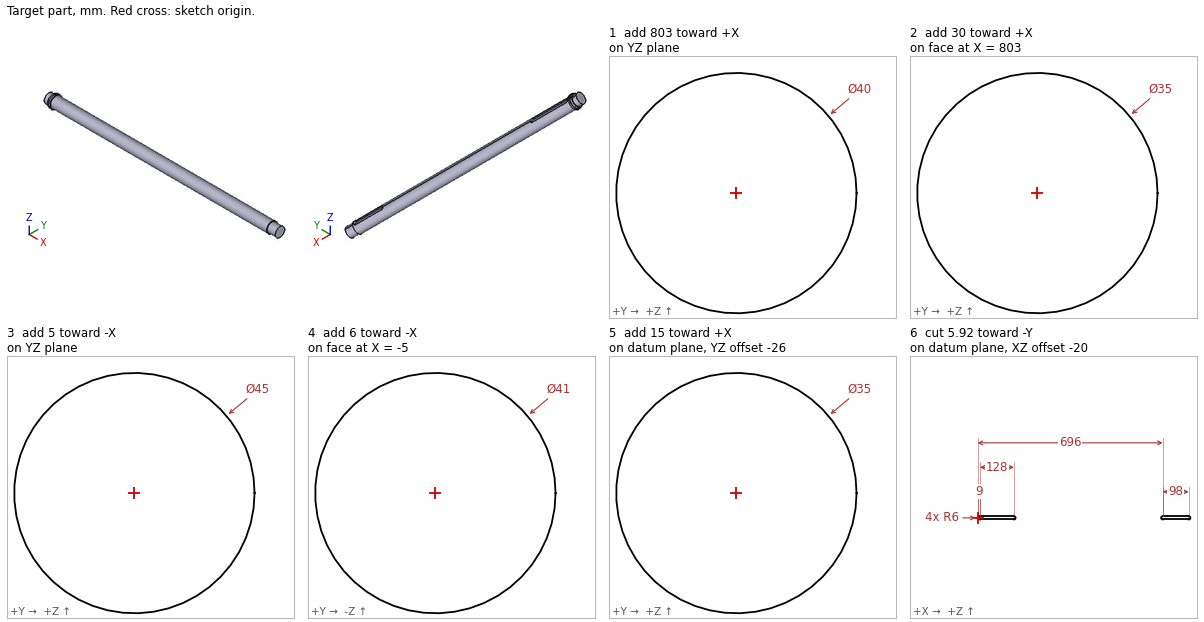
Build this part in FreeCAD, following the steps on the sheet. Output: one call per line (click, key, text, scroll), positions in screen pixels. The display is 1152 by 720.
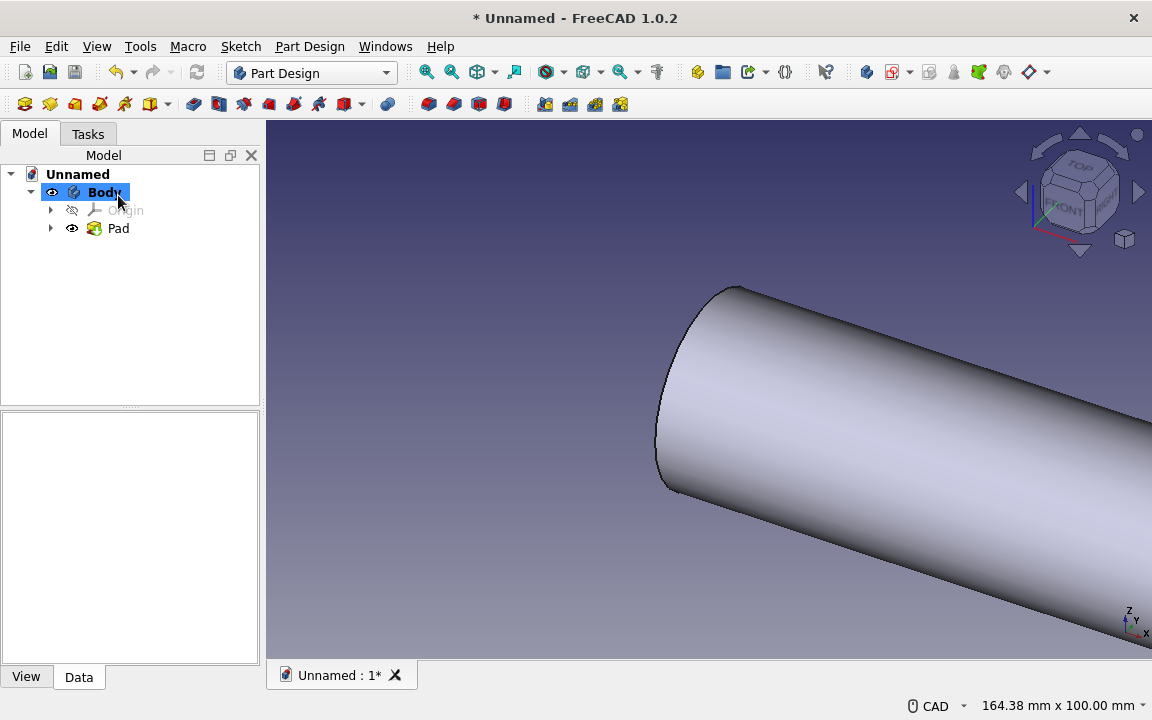
click(427, 72)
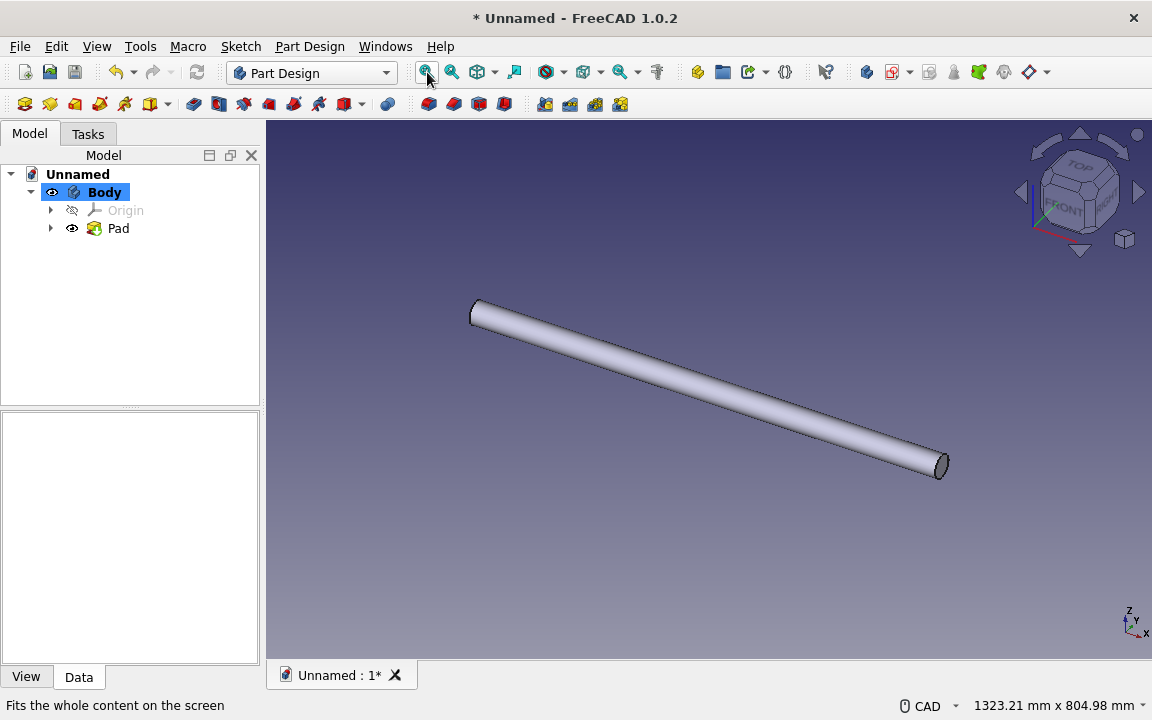
key(0)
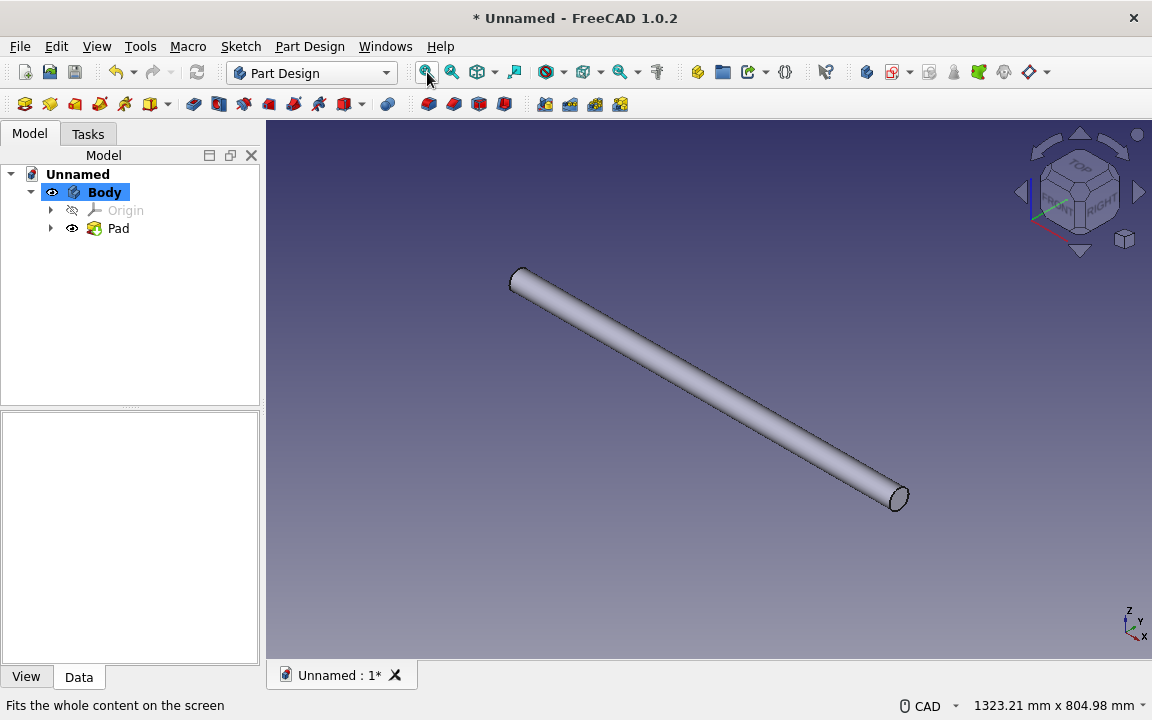
click(902, 497)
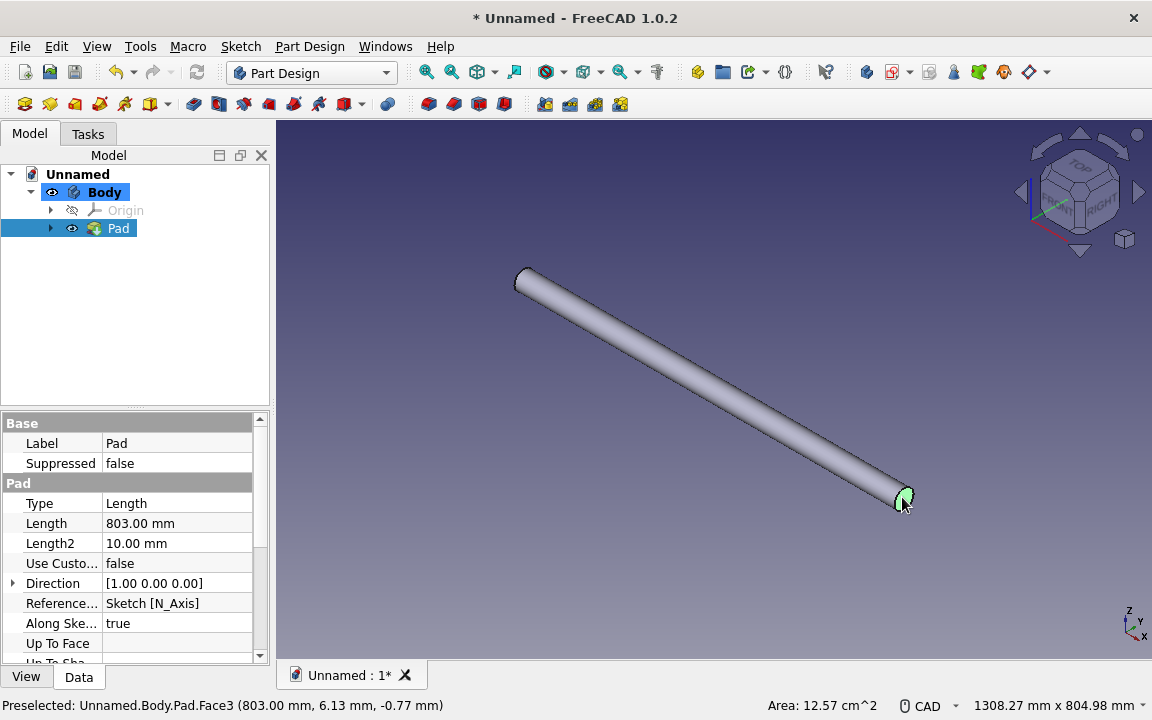
click(892, 72)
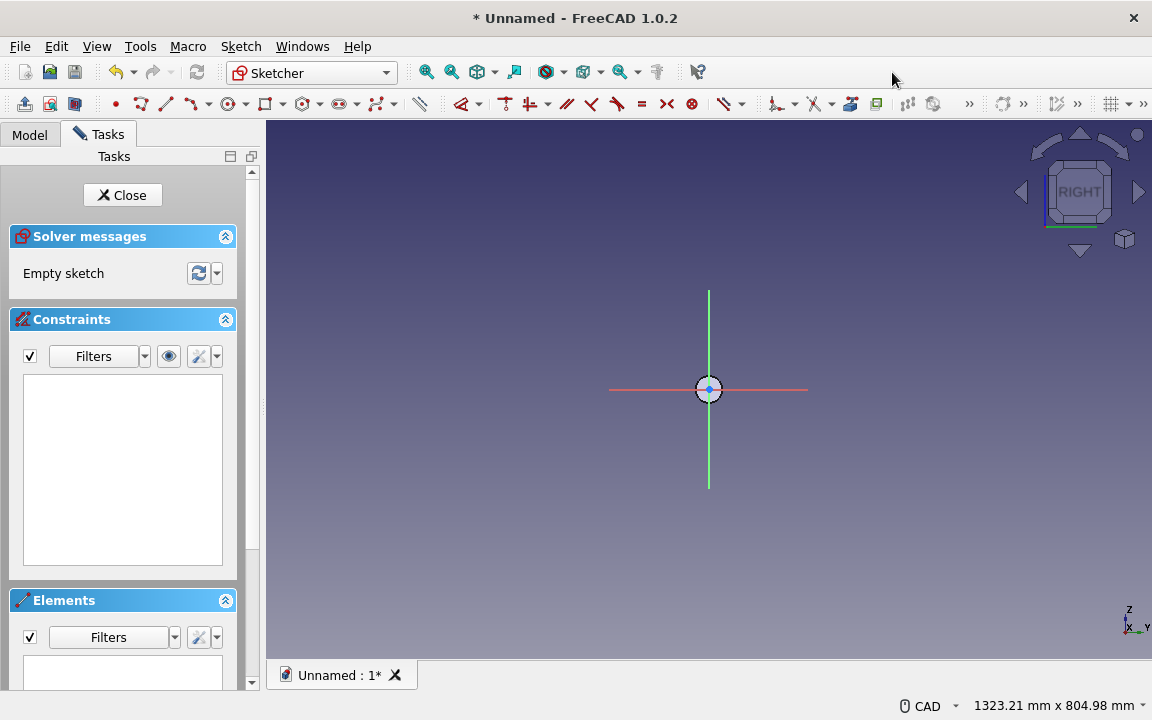
scroll(714, 389, up, 13)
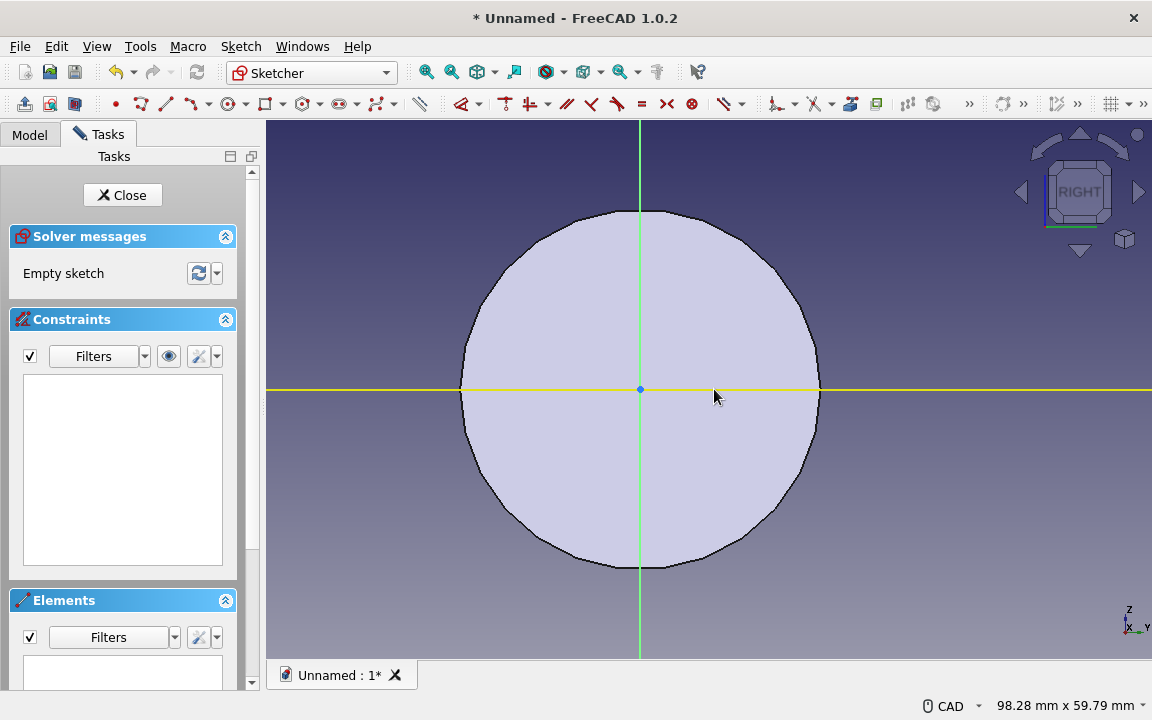
click(228, 104)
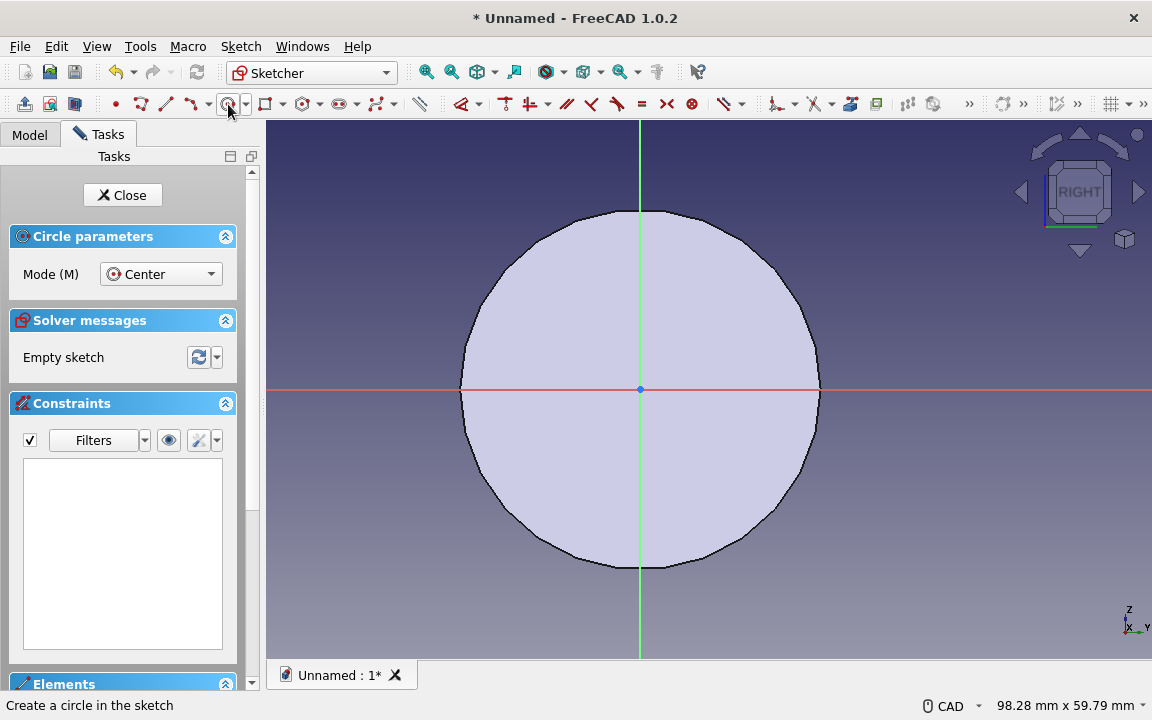
click(640, 389)
move(752, 278)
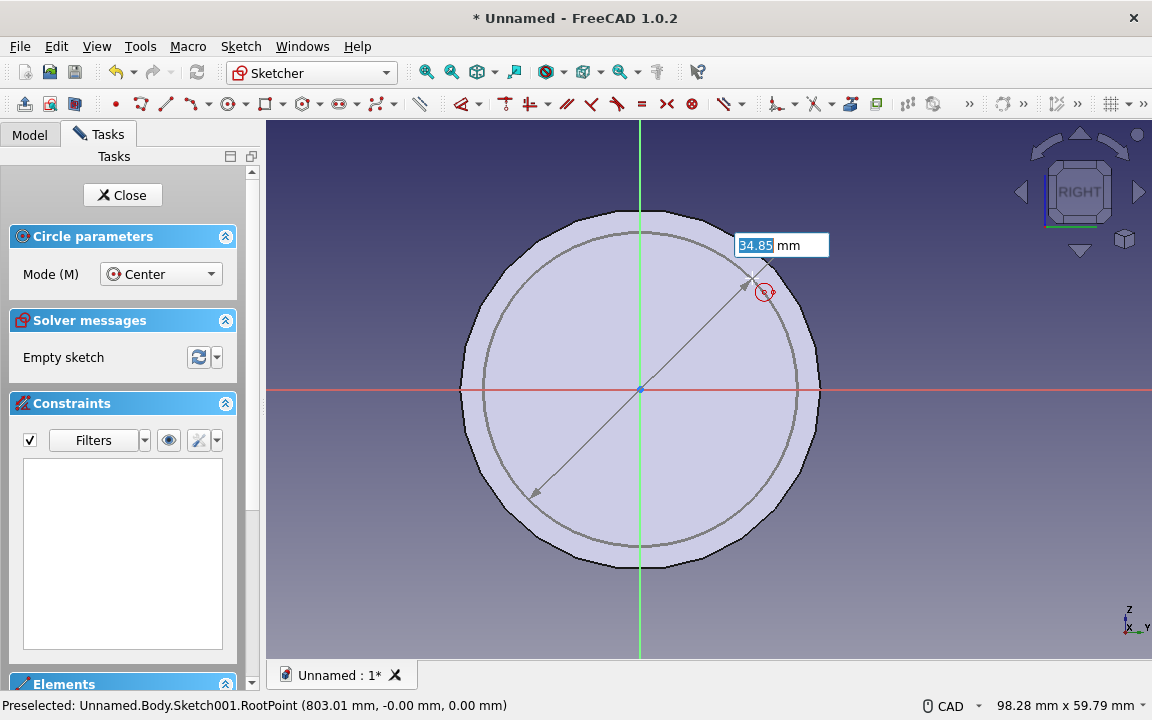
text(35)
key(Return)
key(Escape)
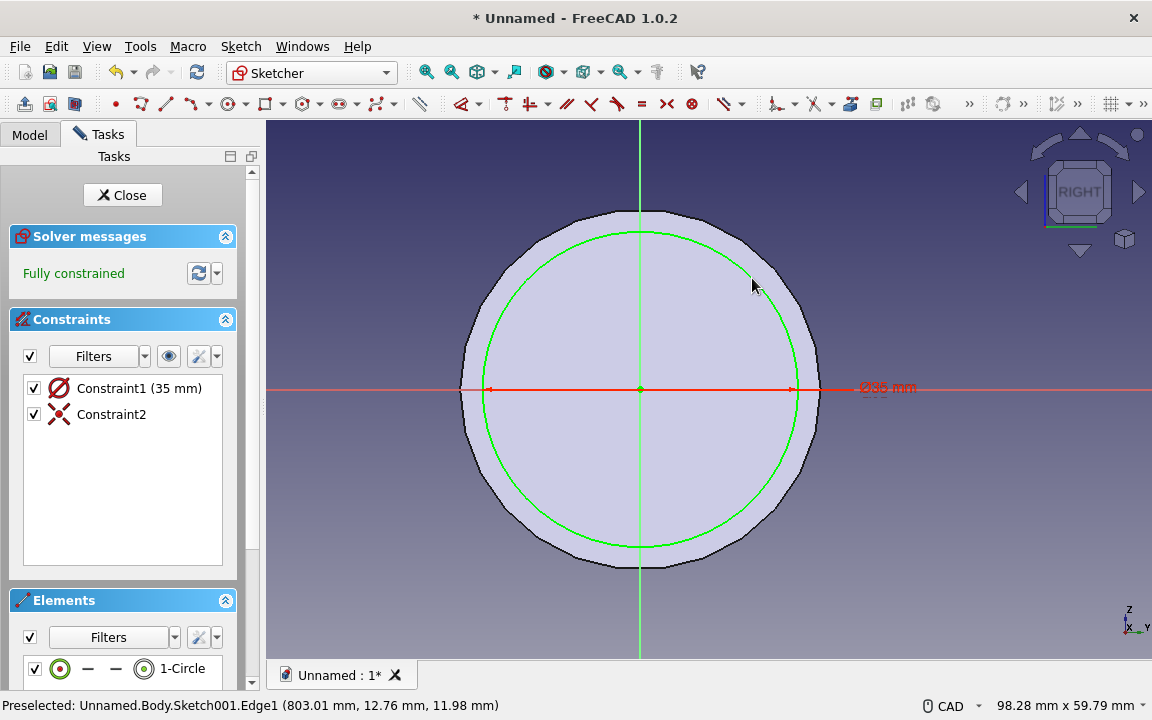
click(123, 195)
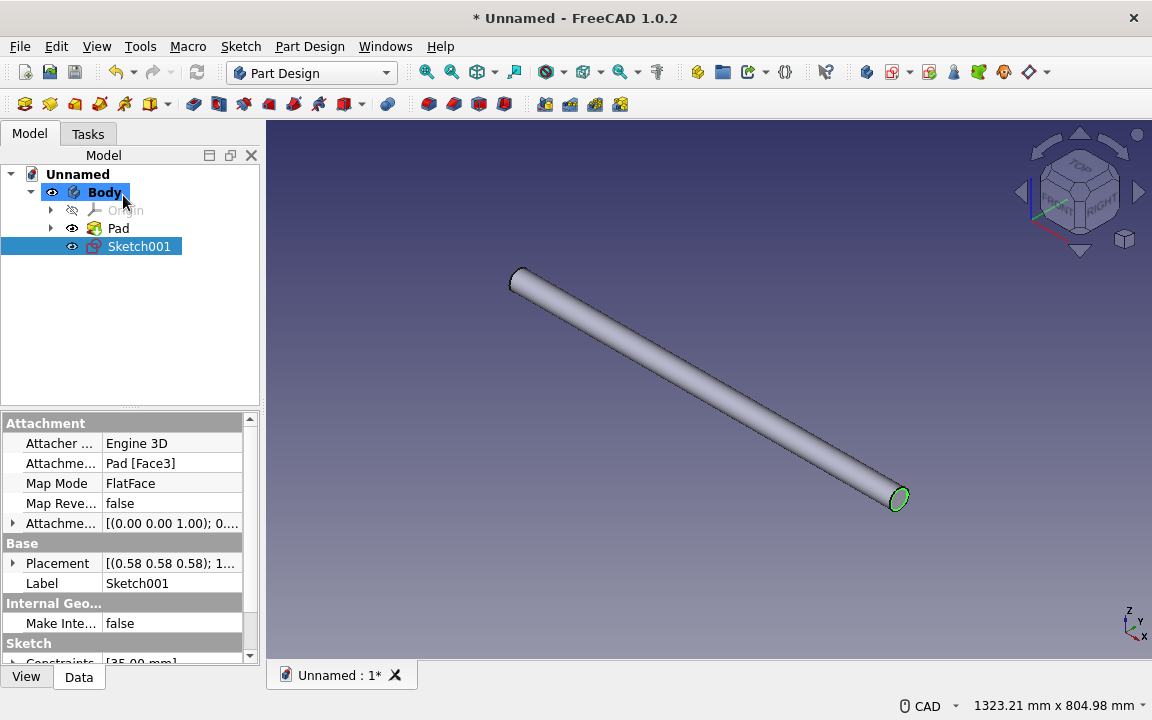
click(25, 104)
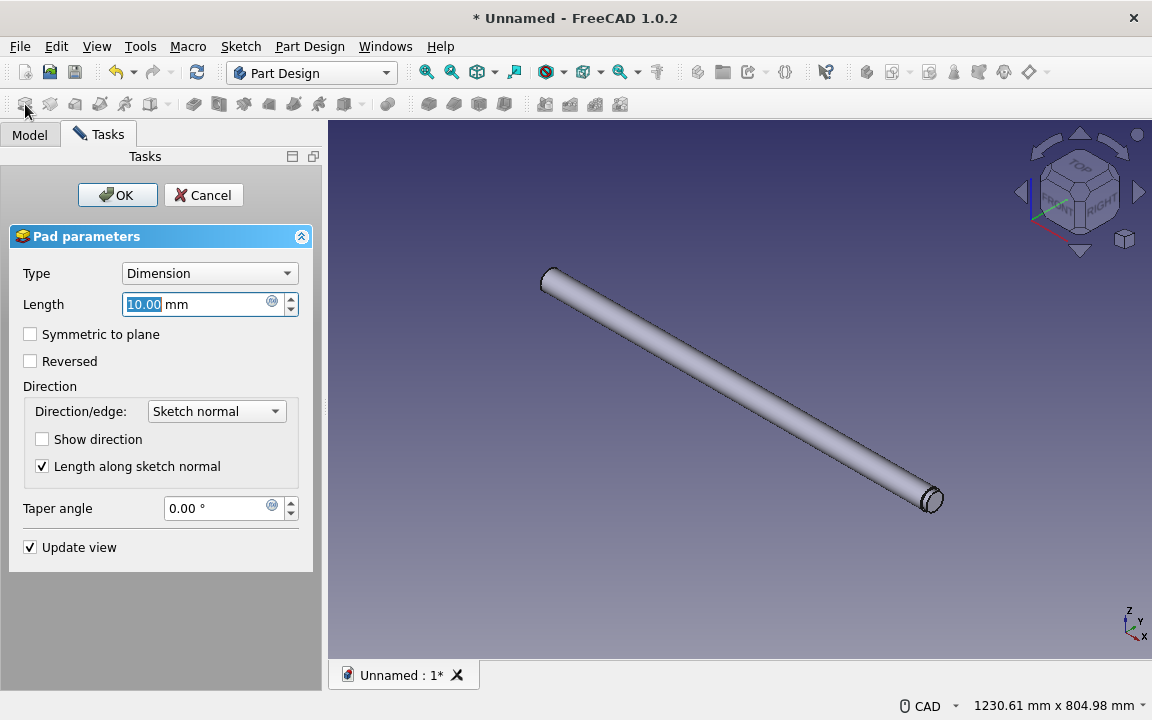
text(30)
key(Tab)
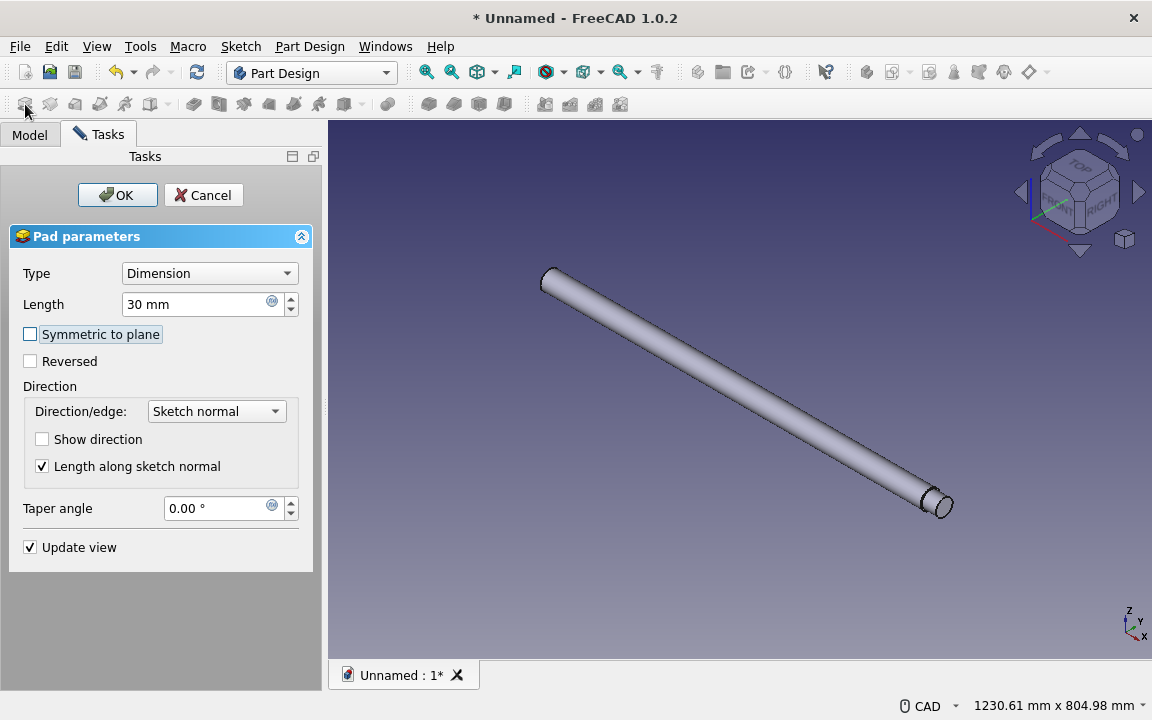
click(118, 195)